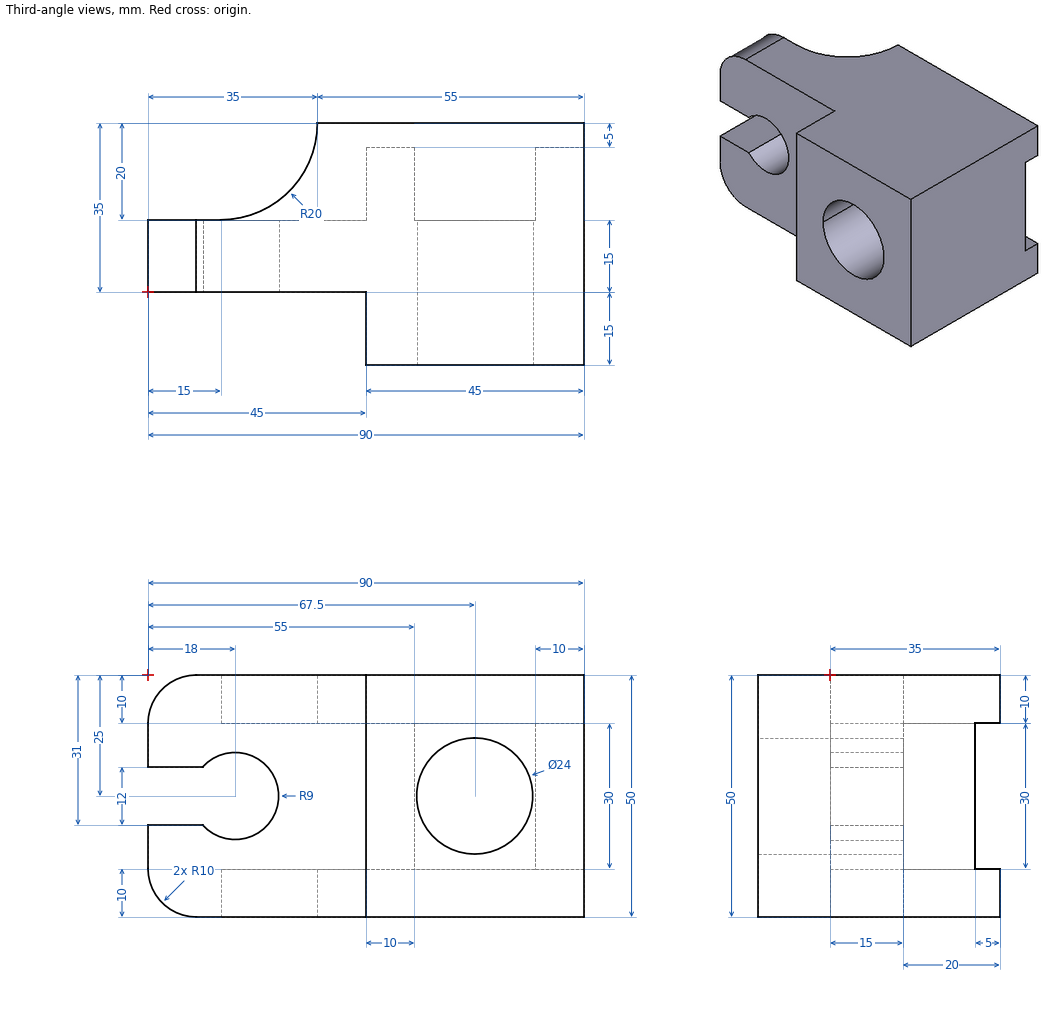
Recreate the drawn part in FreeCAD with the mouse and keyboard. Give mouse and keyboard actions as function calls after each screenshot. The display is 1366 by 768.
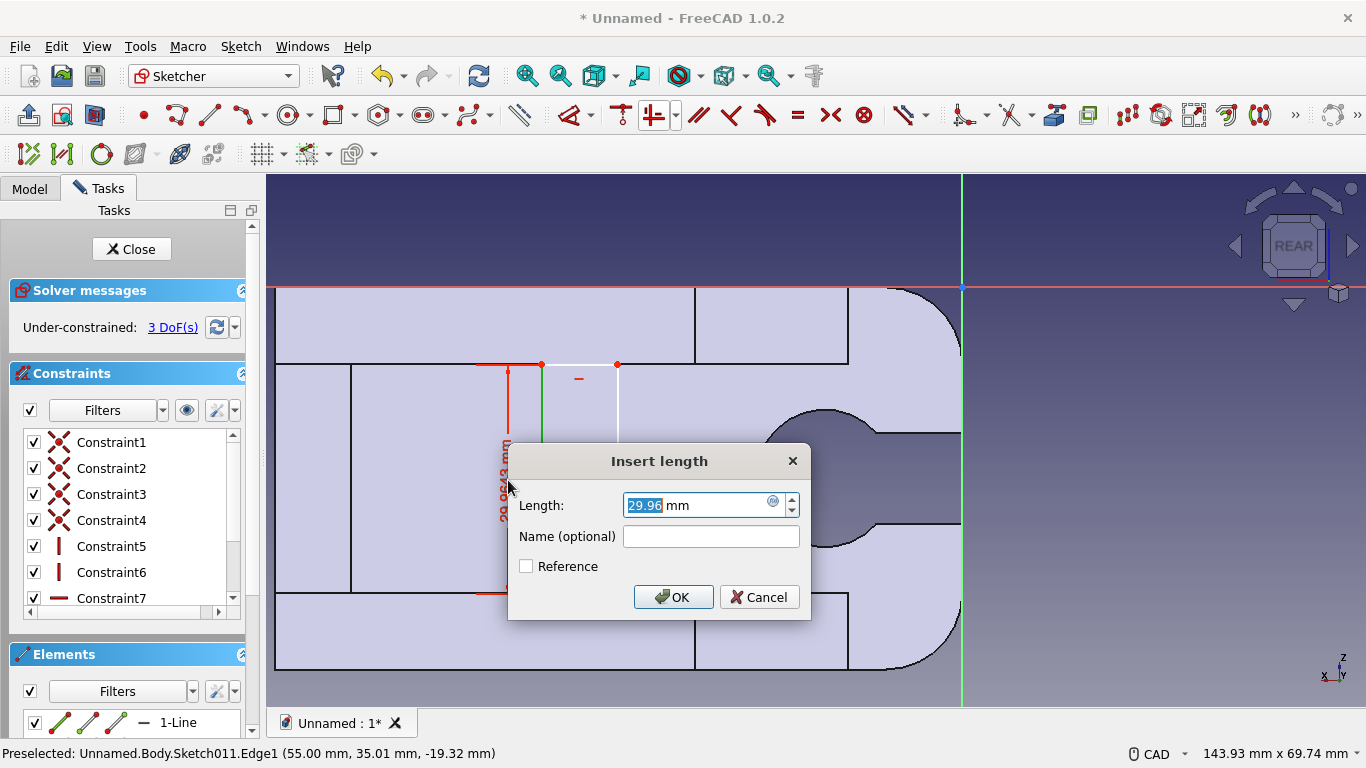
text(30)
key(Return)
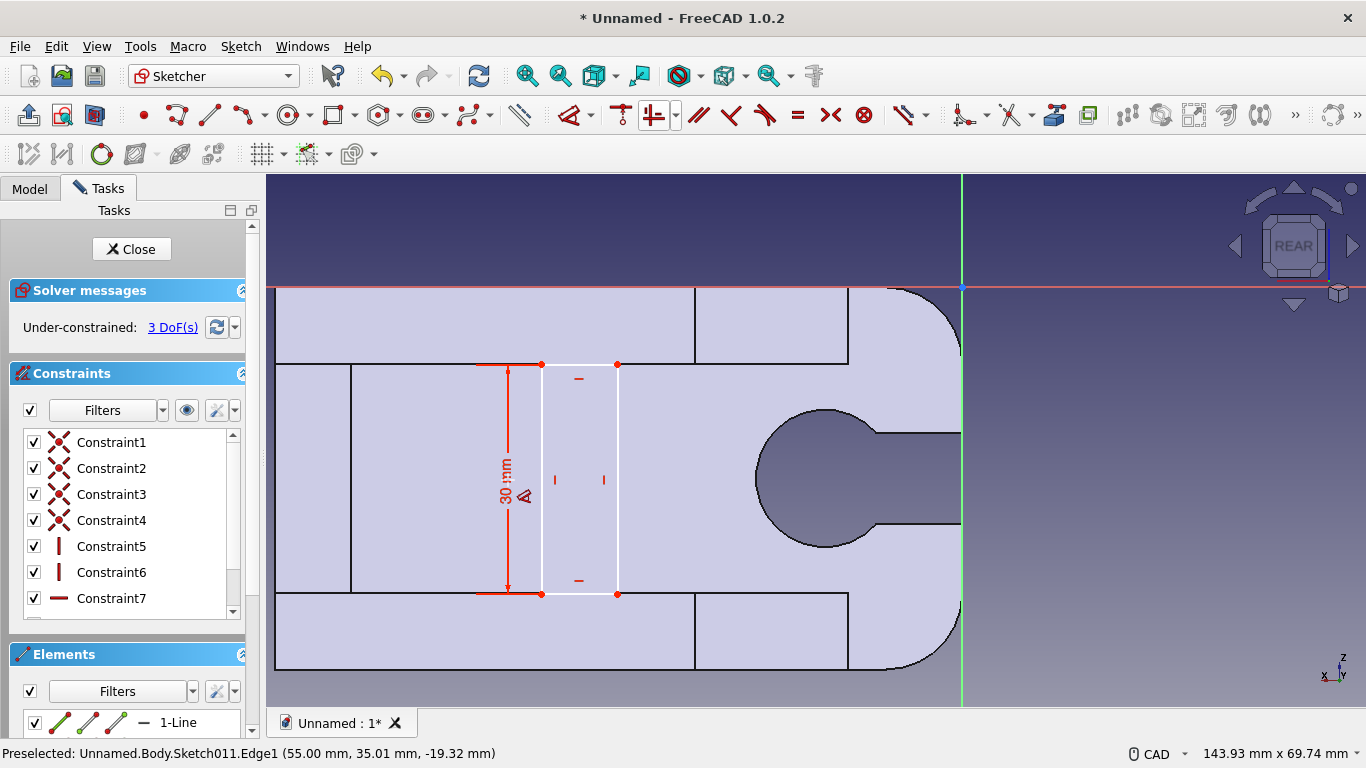
click(565, 594)
click(580, 628)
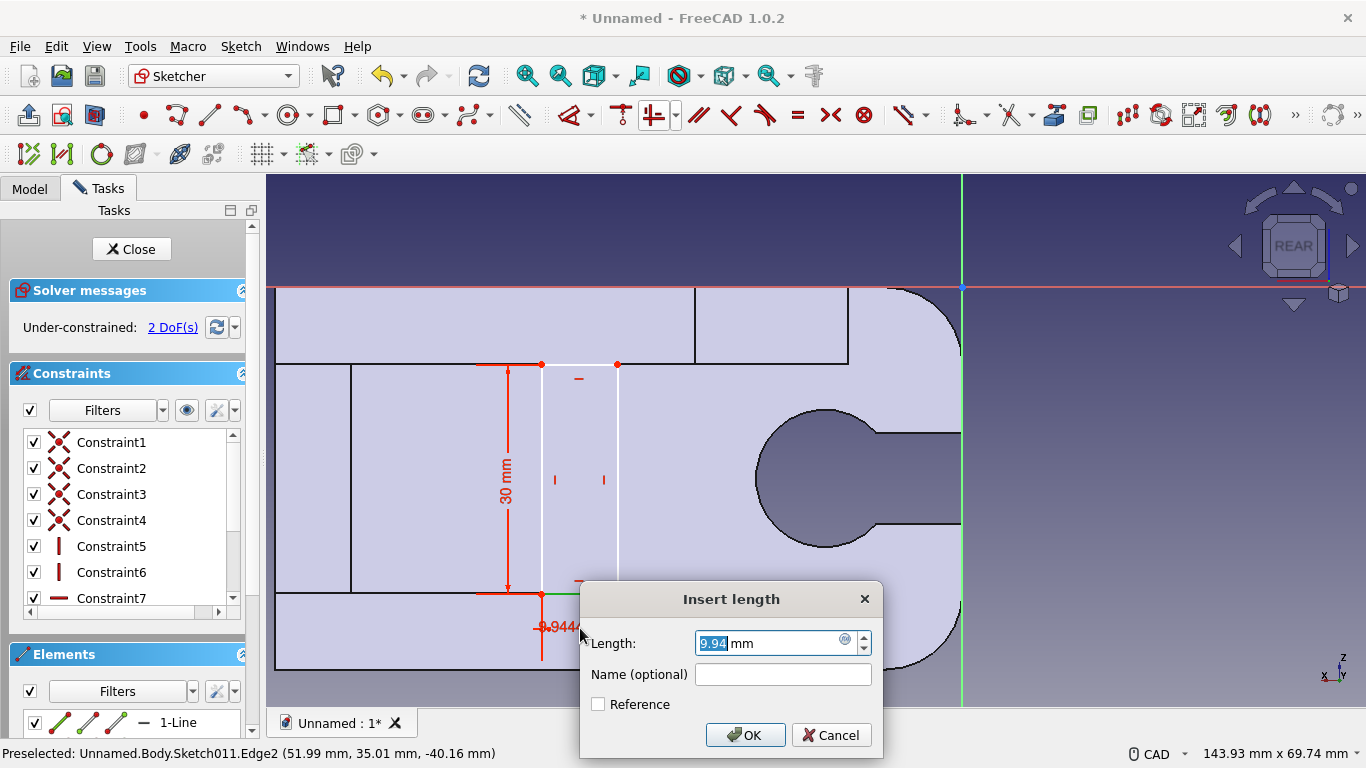
text(10)
key(Return)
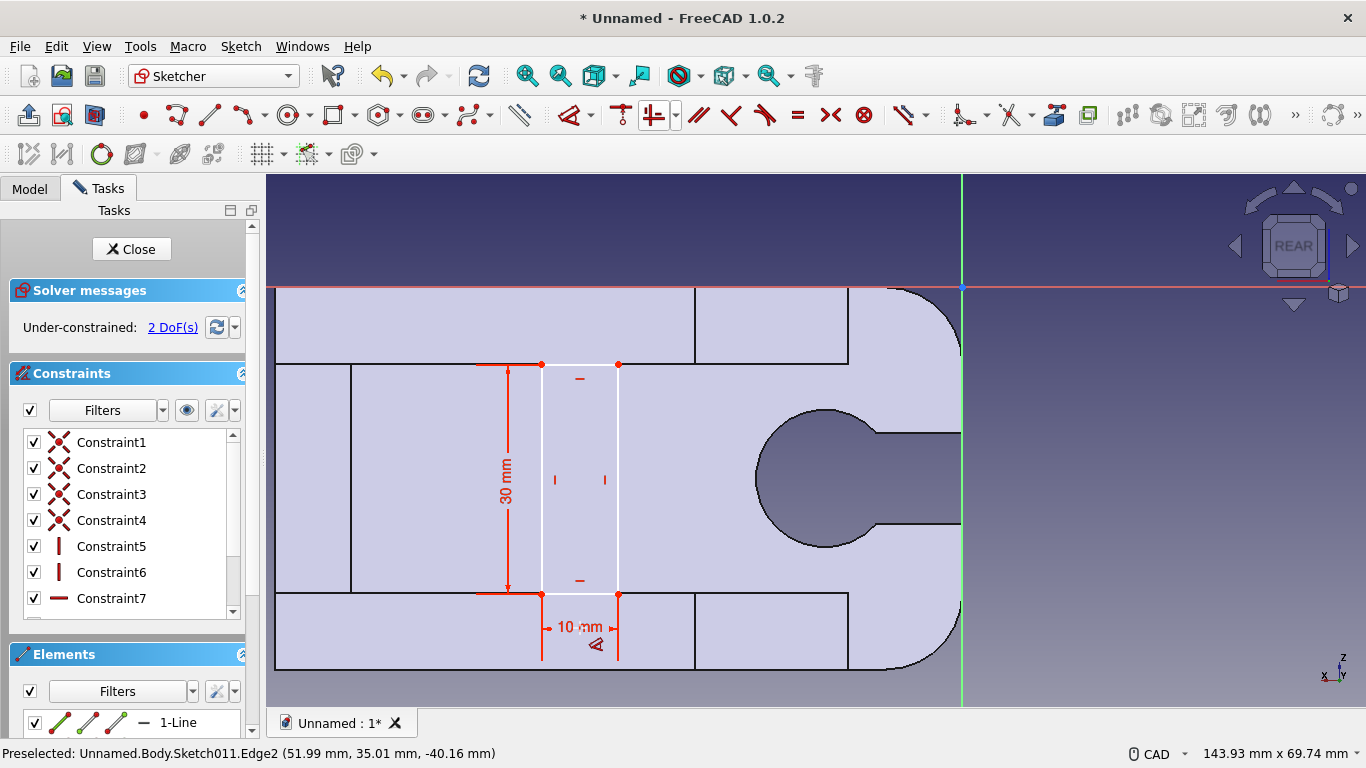
click(542, 365)
click(752, 253)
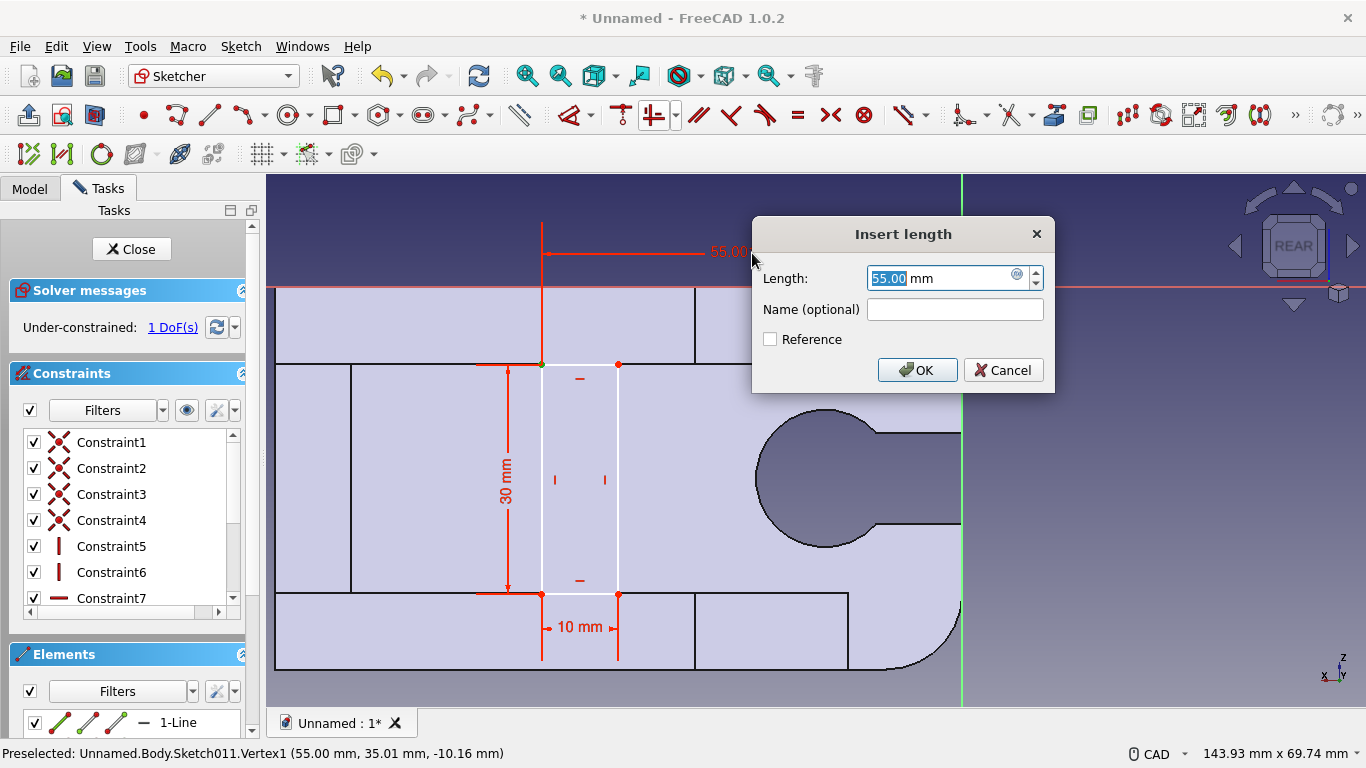
text(55)
key(Return)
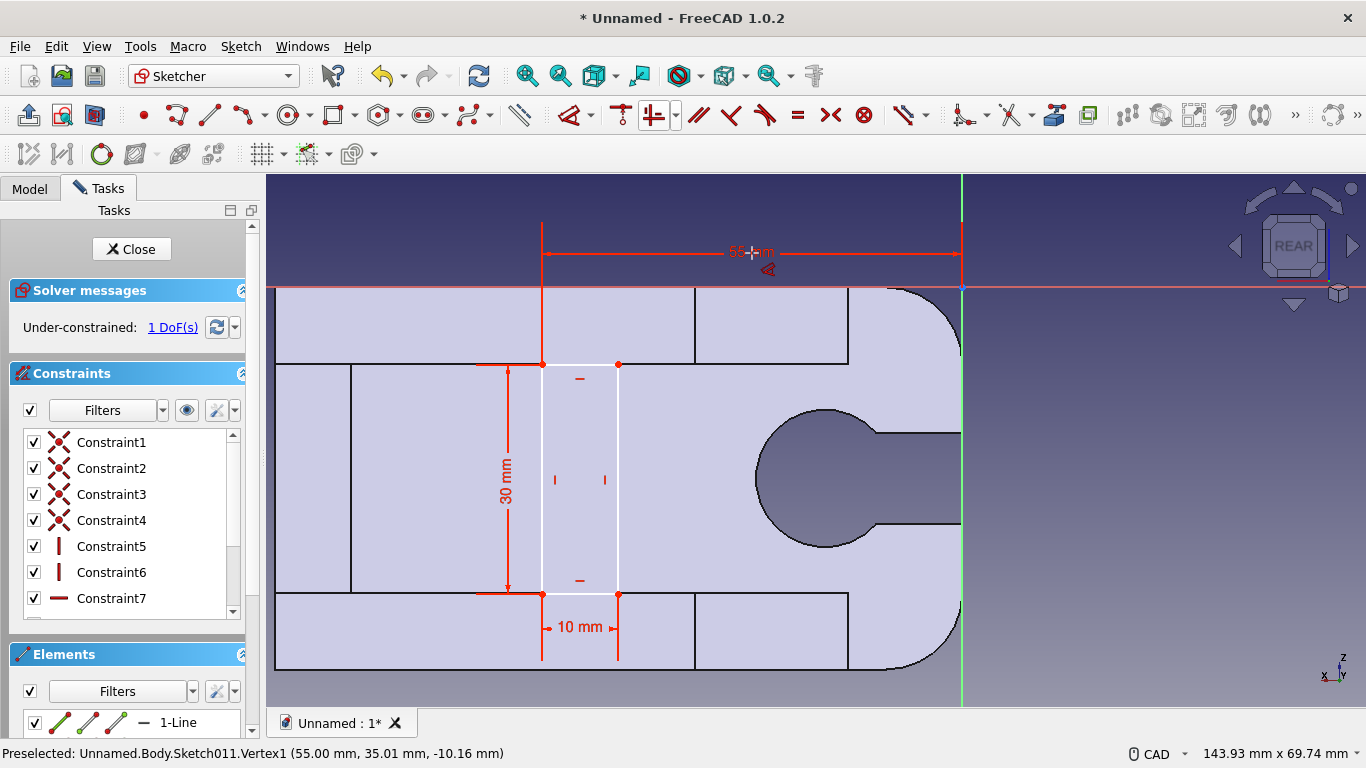
click(542, 365)
click(996, 326)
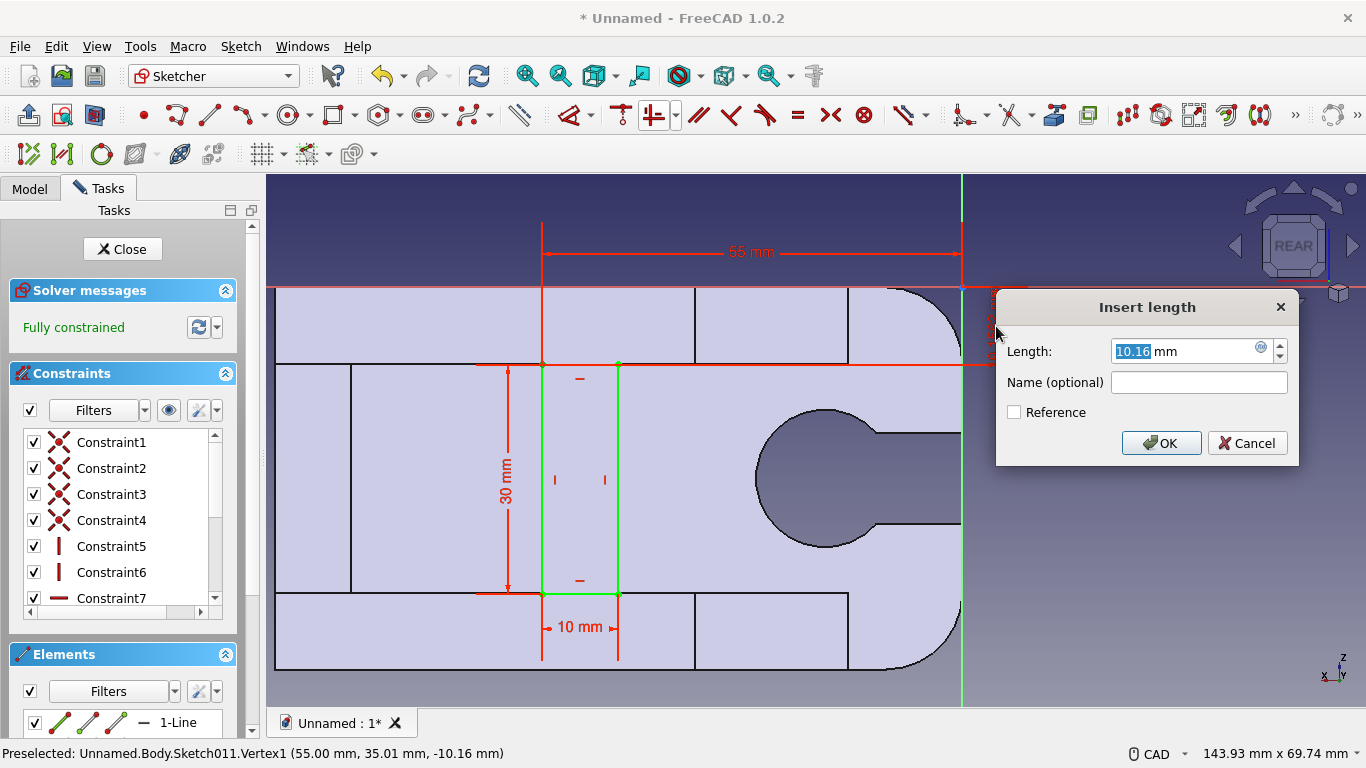
text(10)
key(Return)
key(Escape)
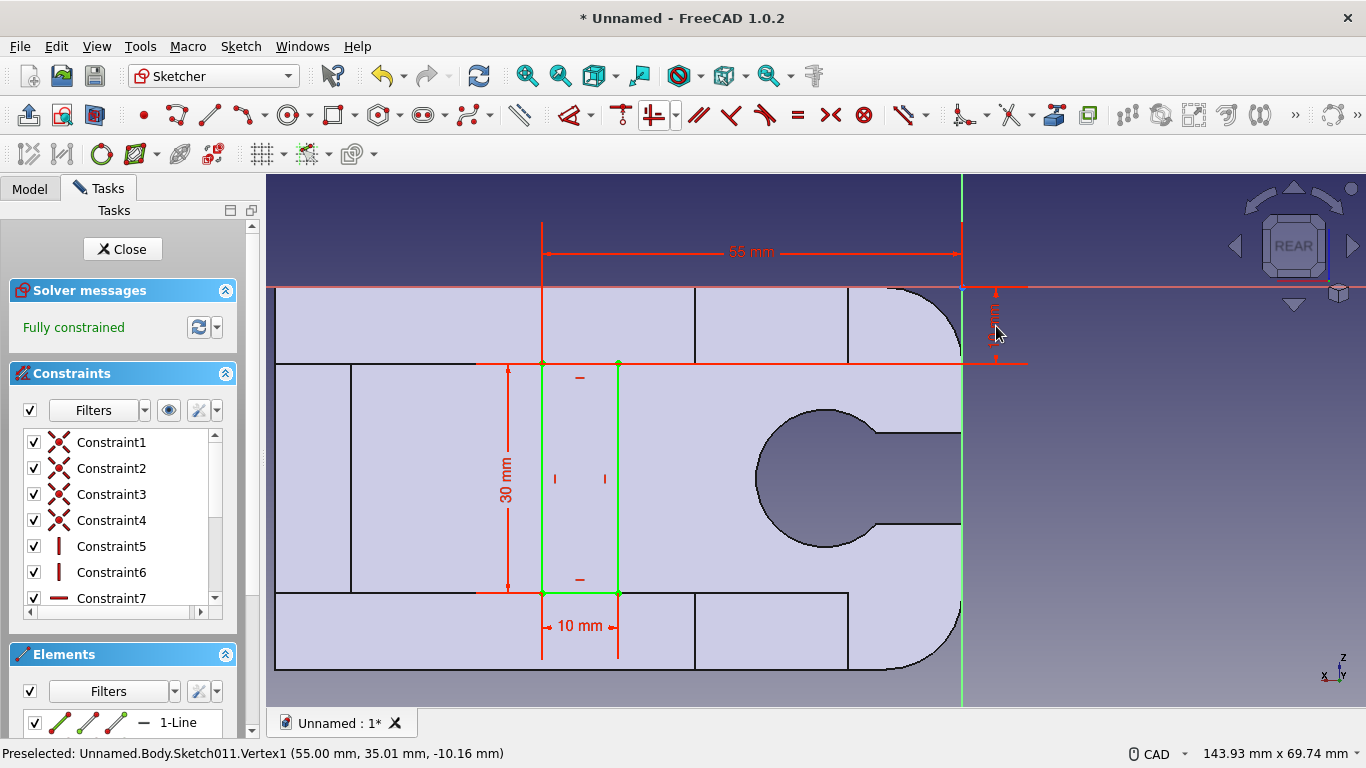
click(123, 249)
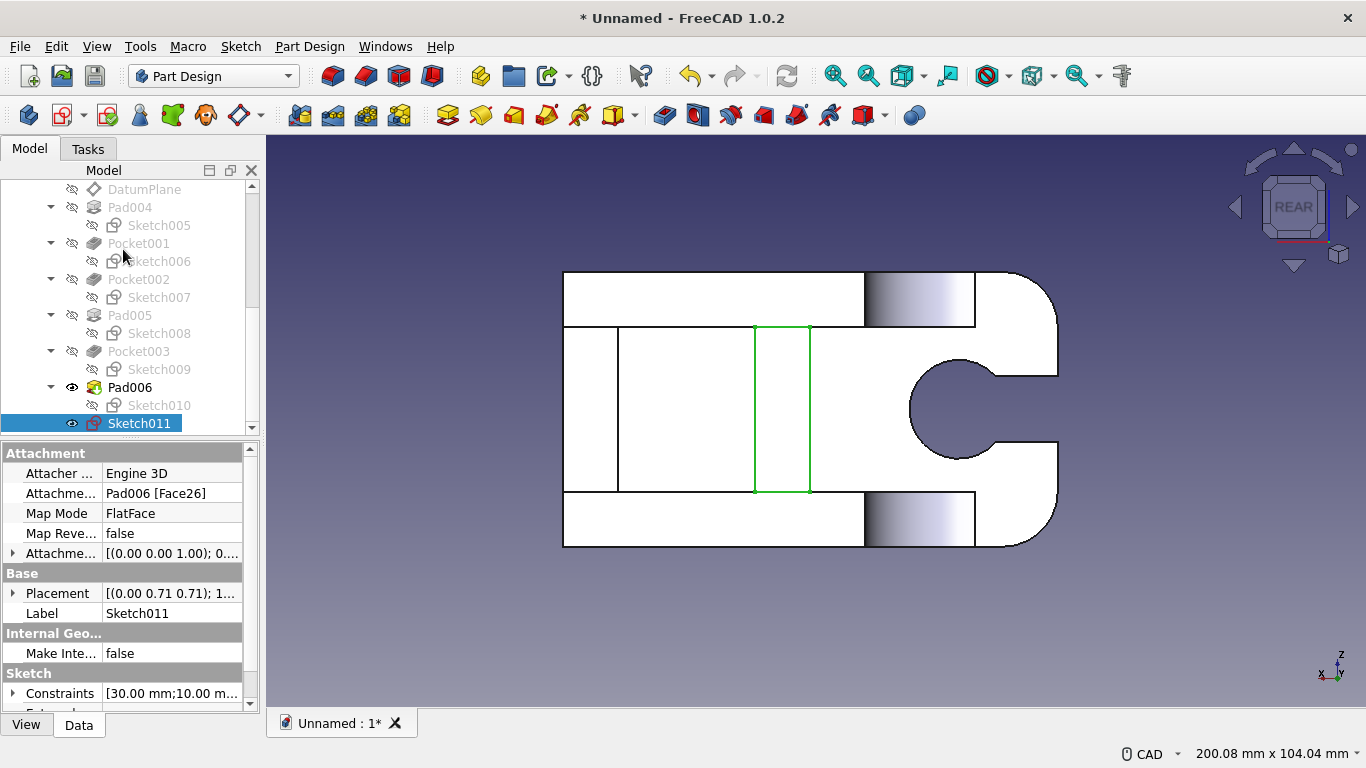
click(665, 116)